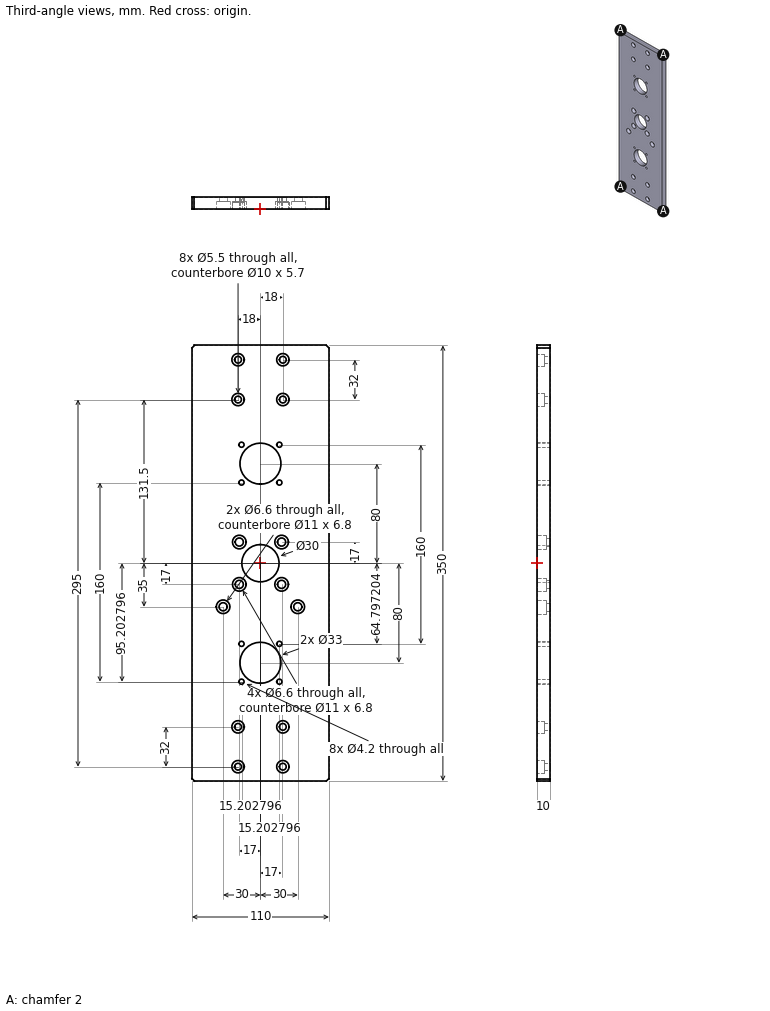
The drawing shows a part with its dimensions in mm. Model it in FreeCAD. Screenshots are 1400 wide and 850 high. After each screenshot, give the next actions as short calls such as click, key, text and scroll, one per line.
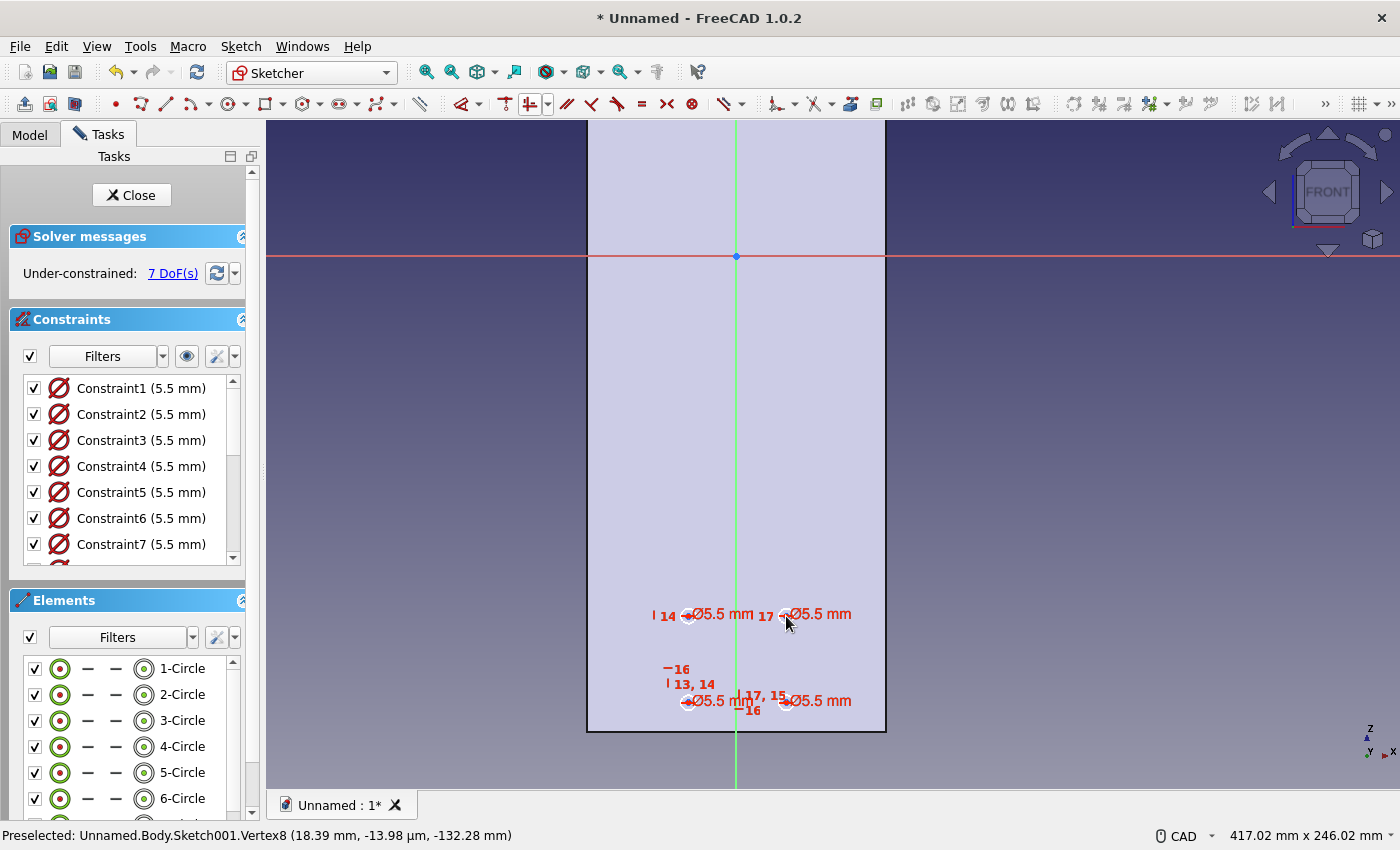
click(689, 616)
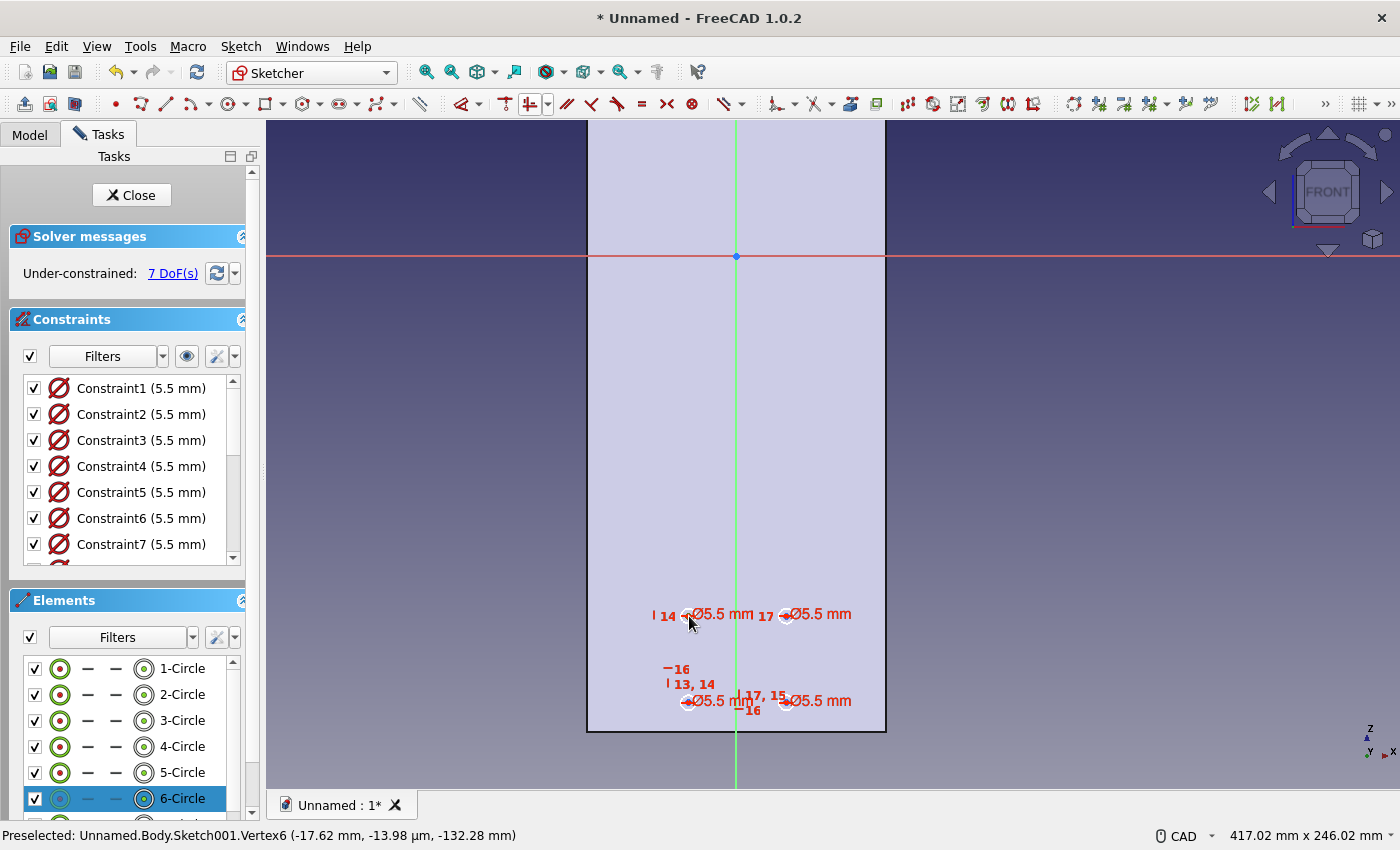
click(786, 616)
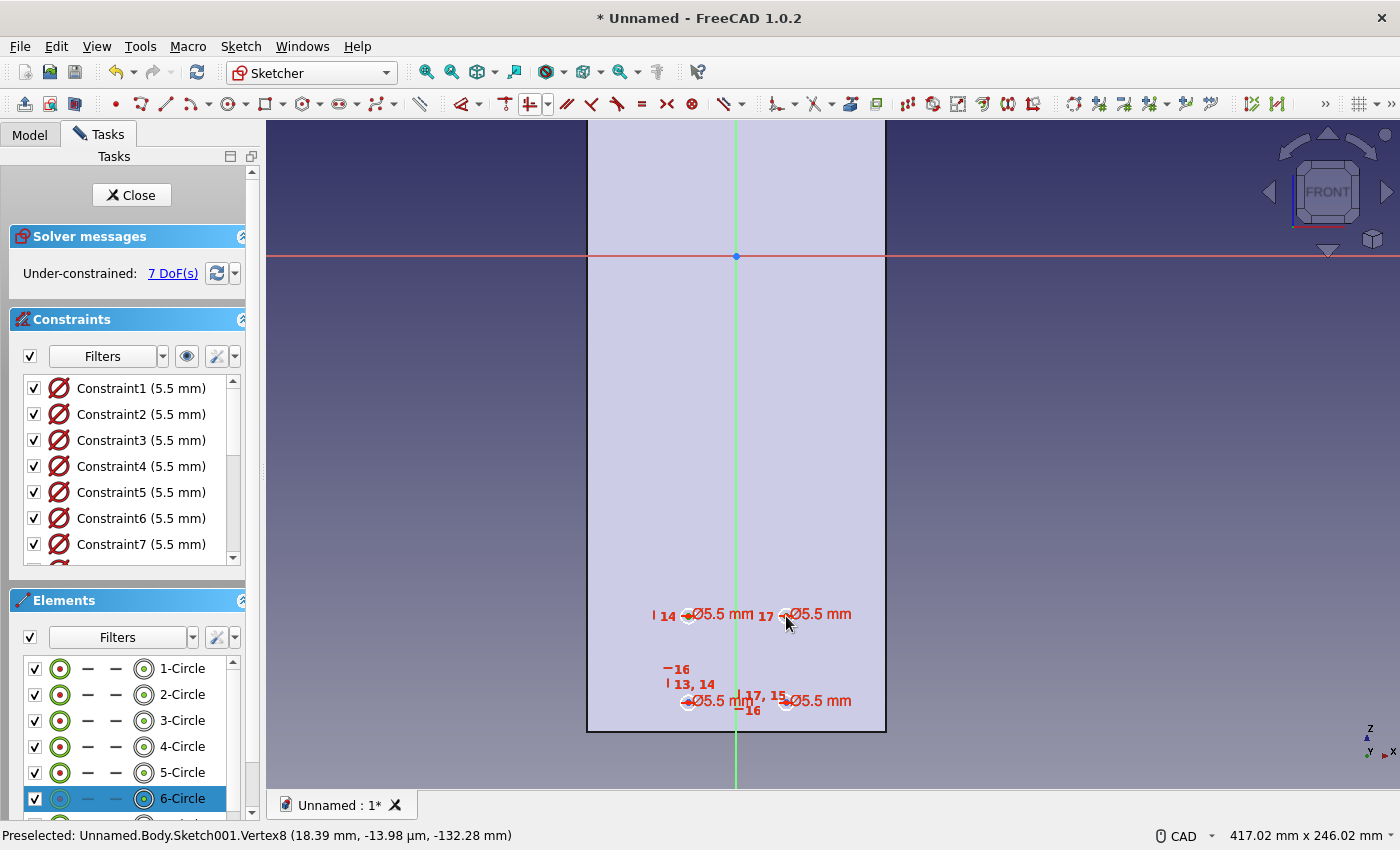
click(548, 104)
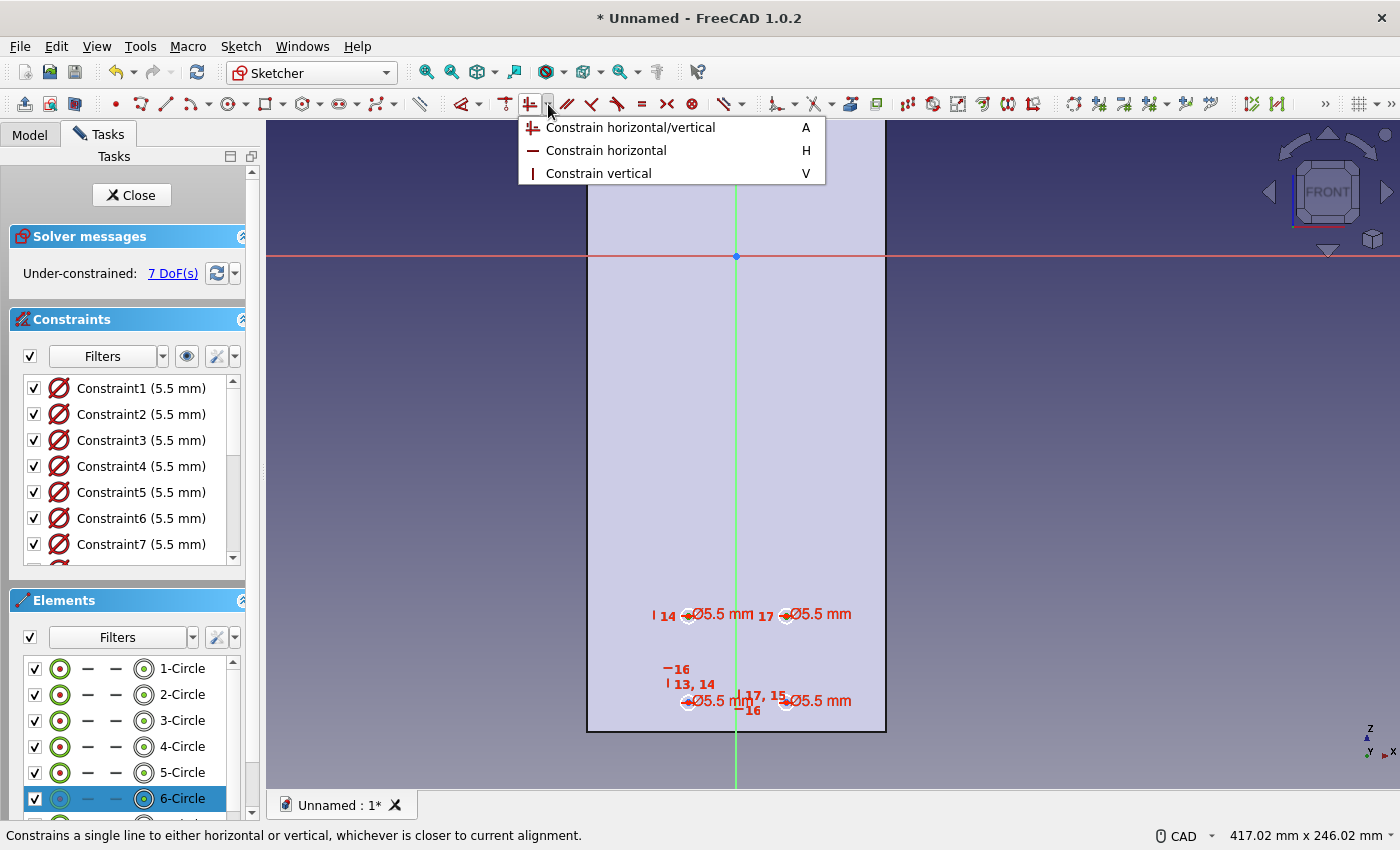
click(672, 150)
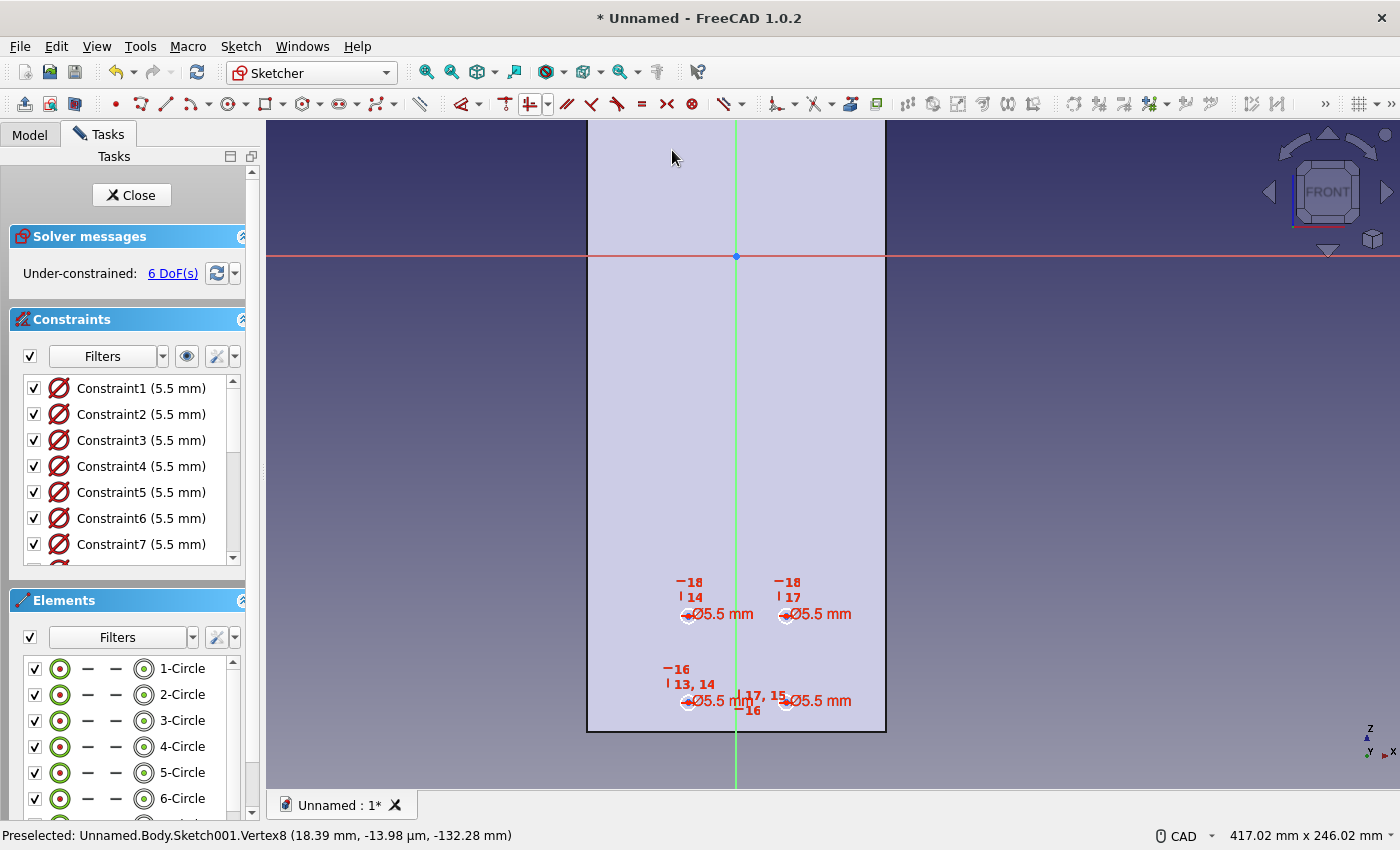
scroll(787, 616, down, 4)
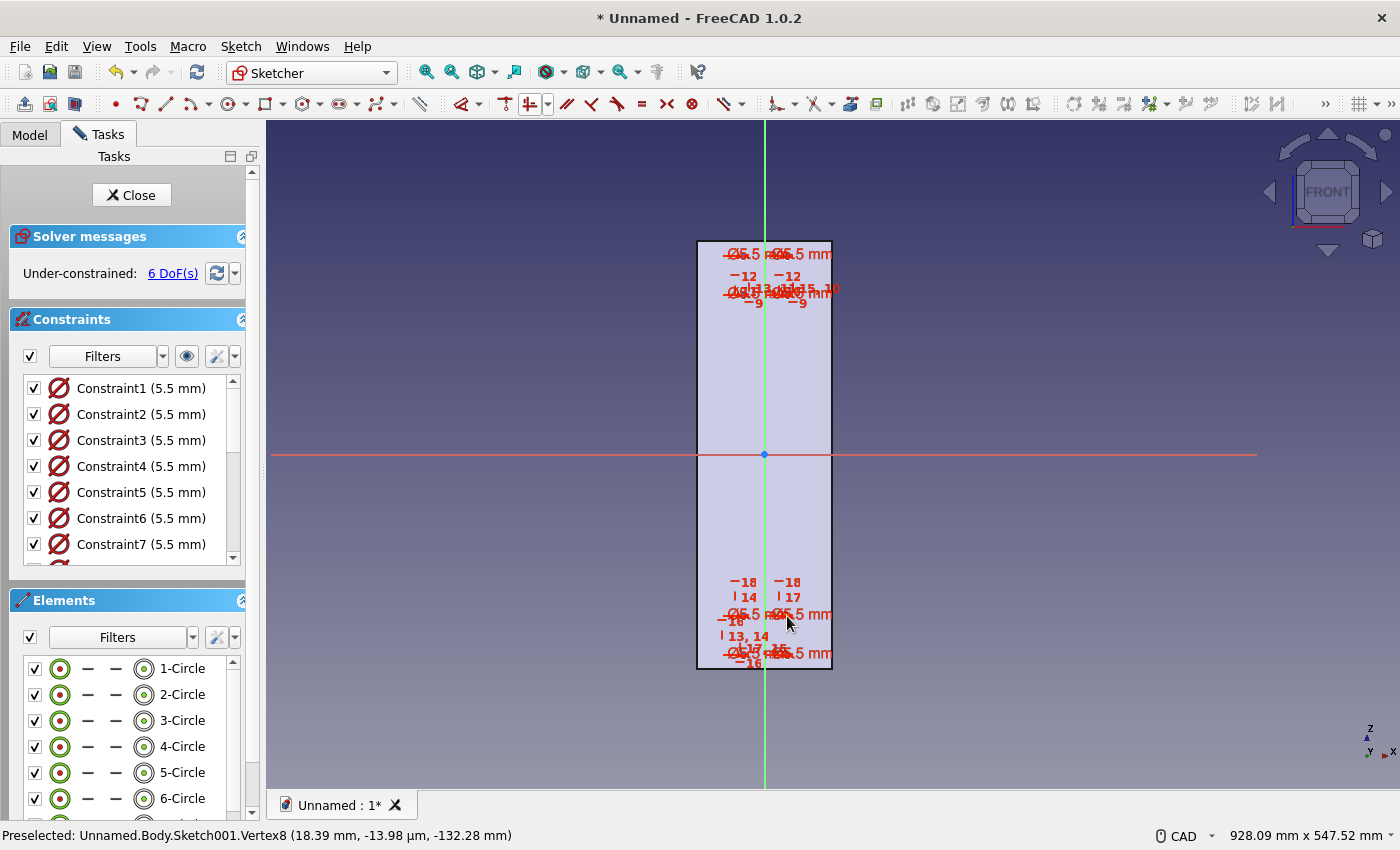
scroll(743, 295, up, 3)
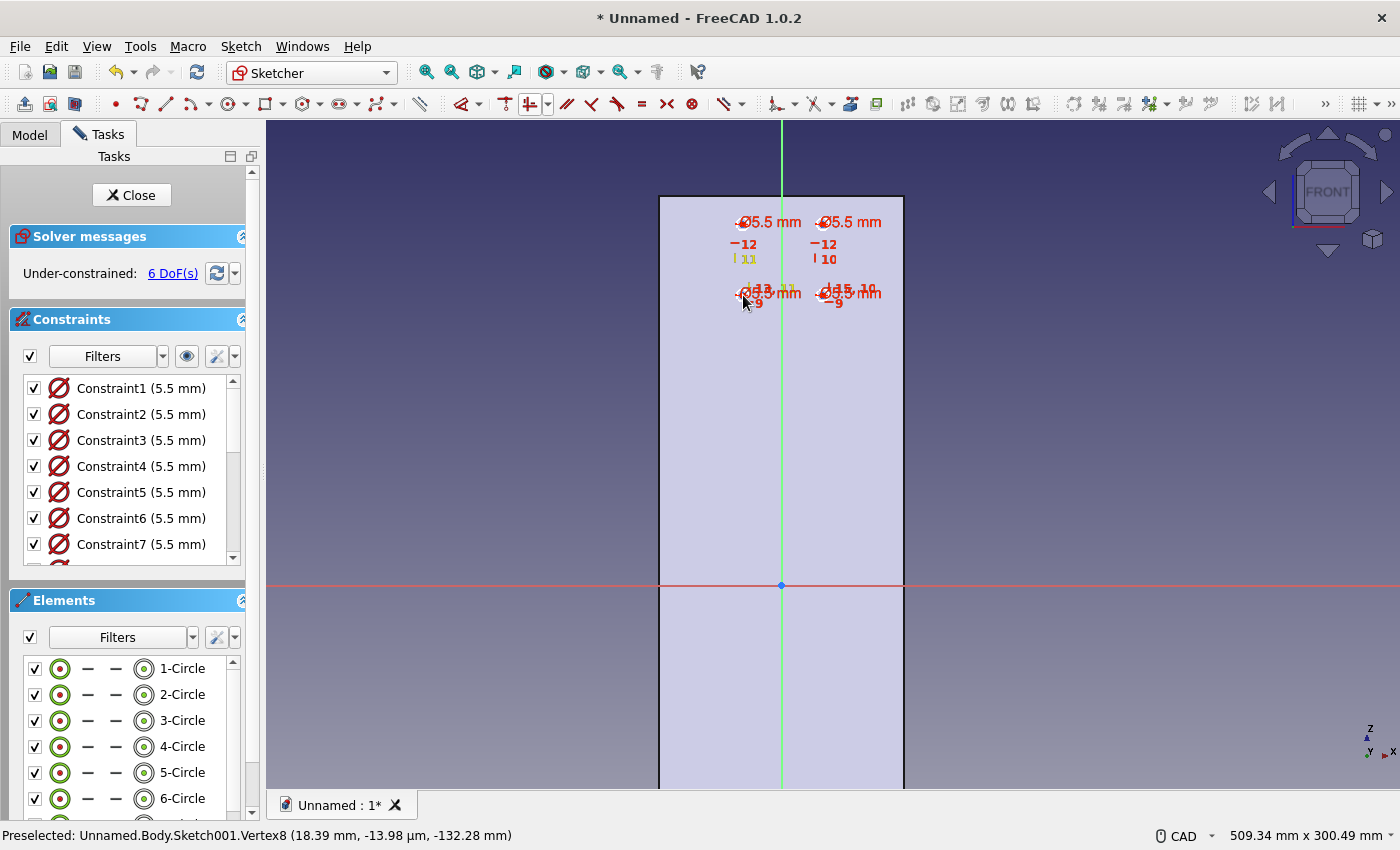
click(743, 295)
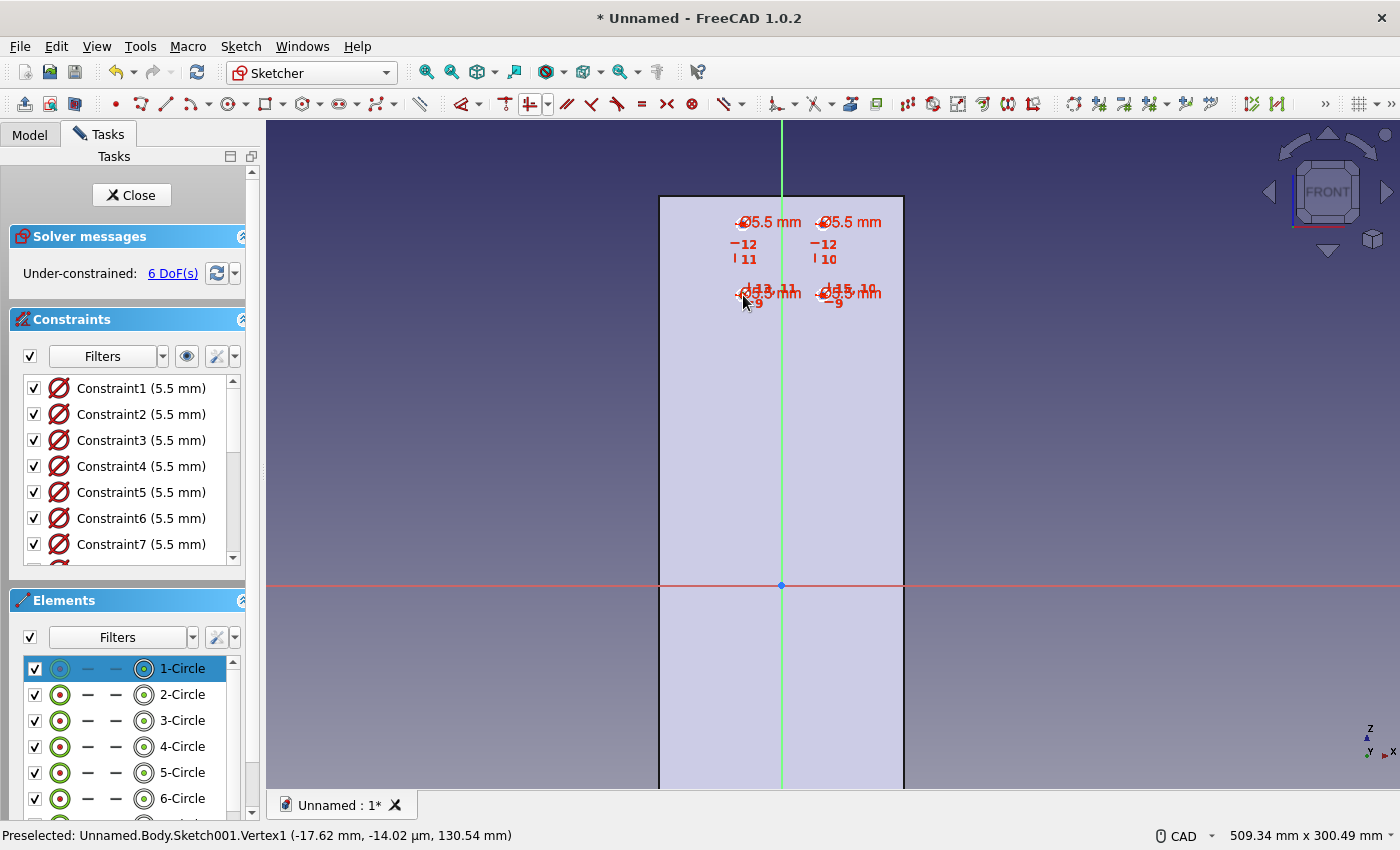
click(478, 104)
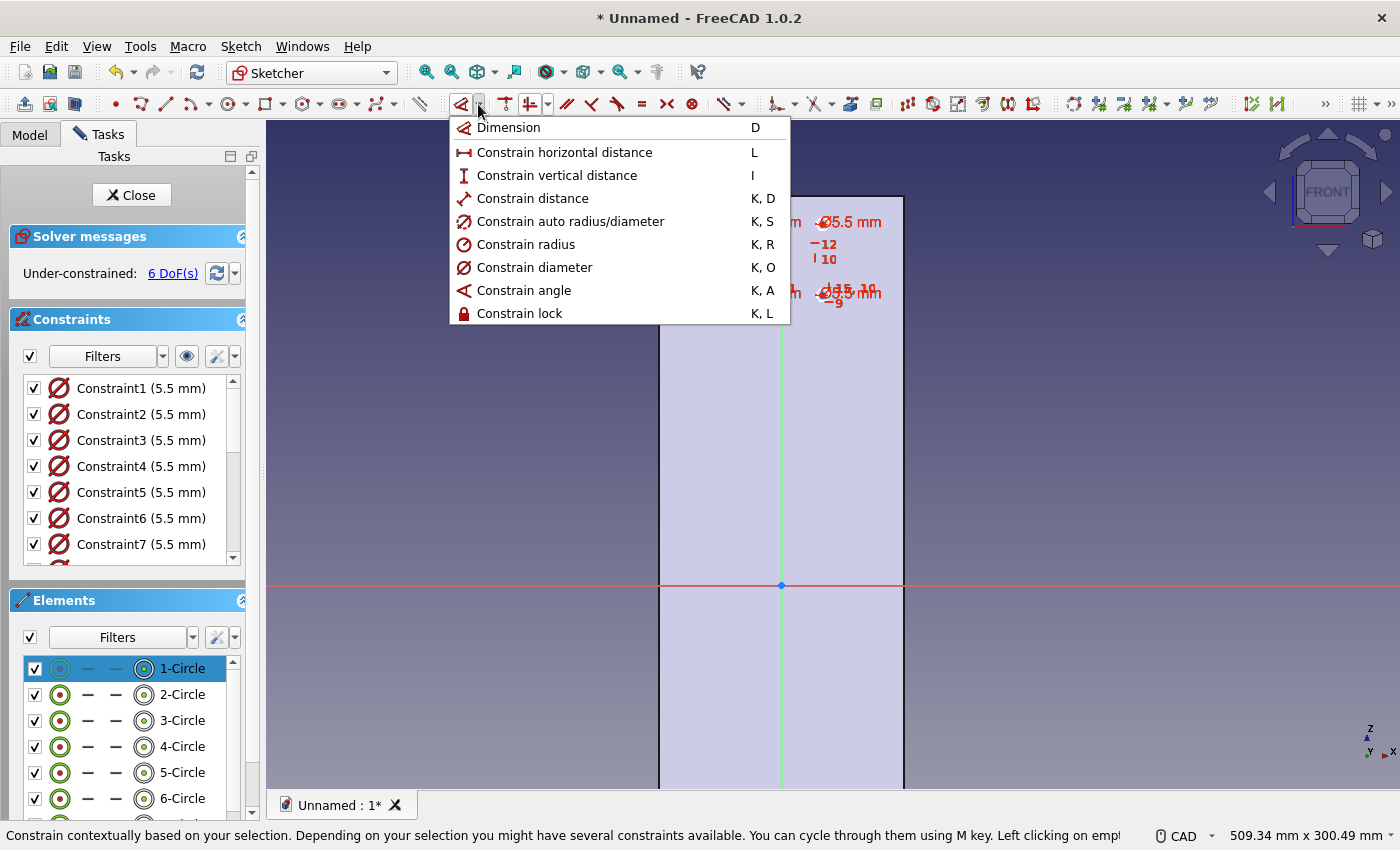
click(620, 152)